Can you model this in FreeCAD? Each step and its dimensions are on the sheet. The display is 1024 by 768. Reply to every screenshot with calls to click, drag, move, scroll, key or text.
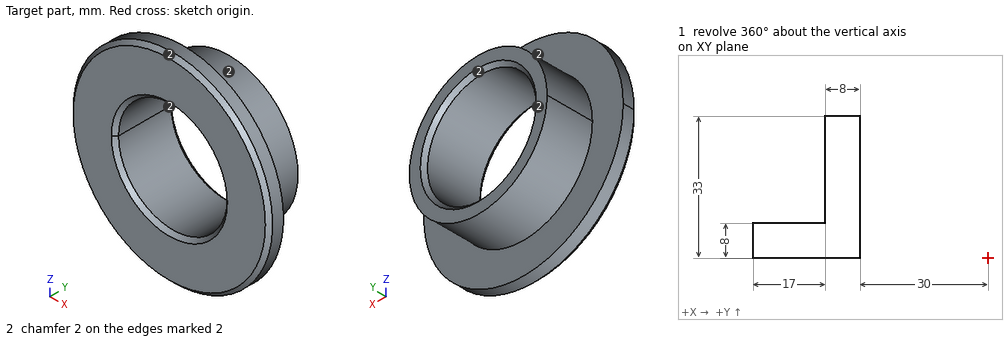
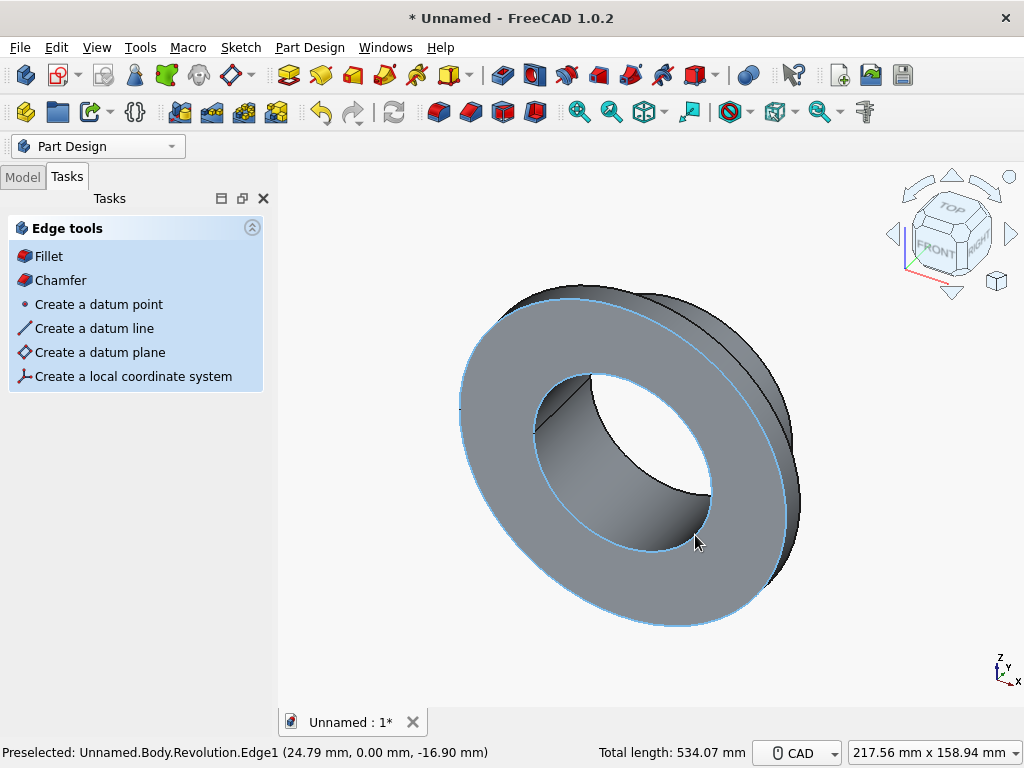
key(0)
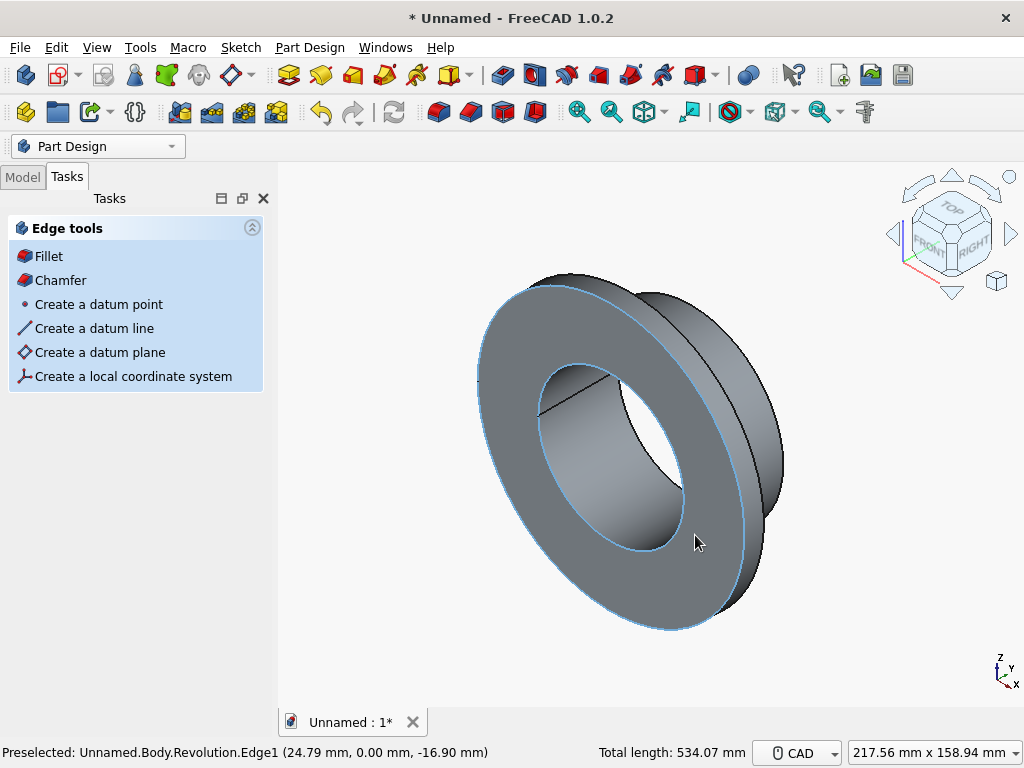
key(2)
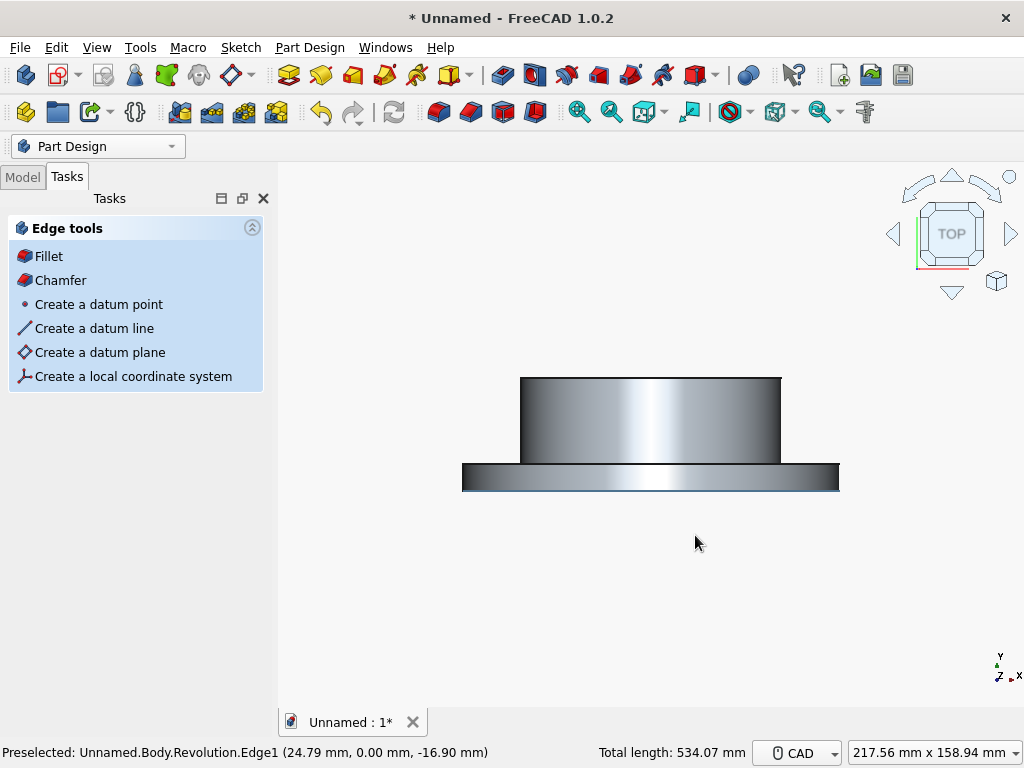
key(1)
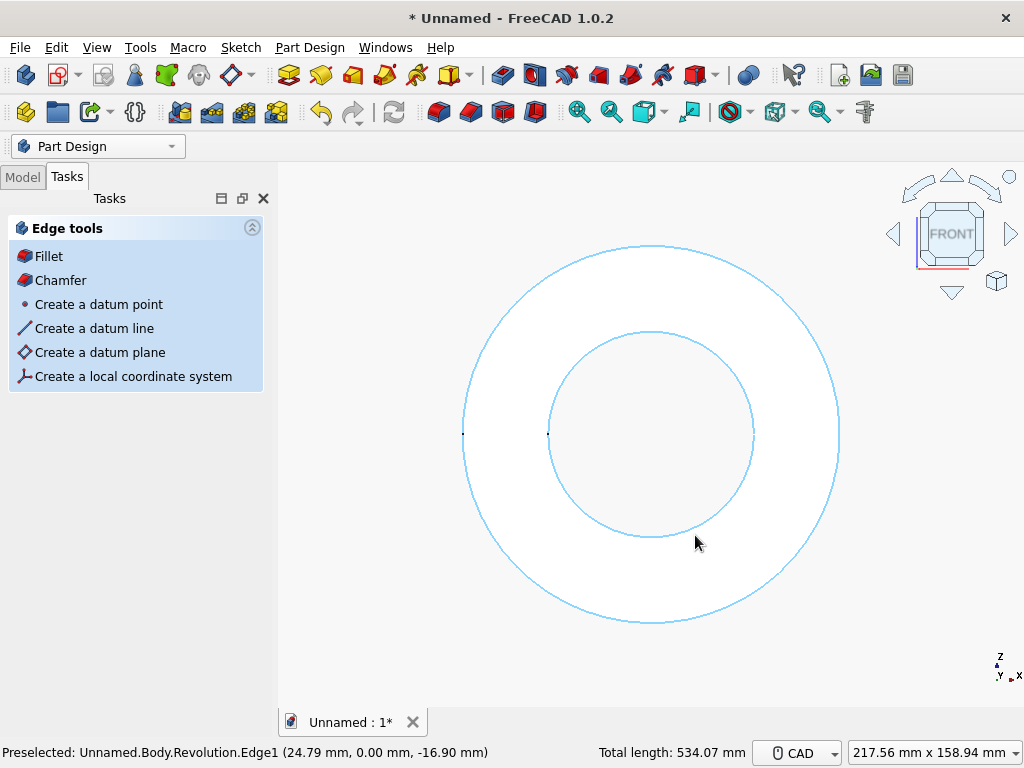
key(3)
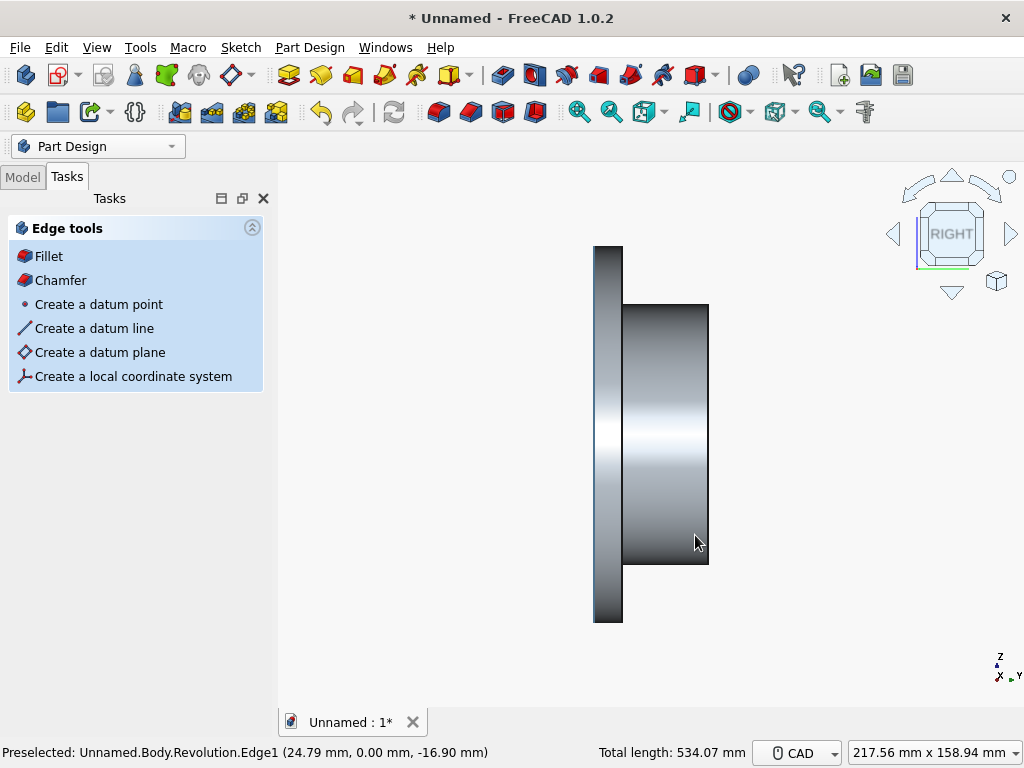
key(5)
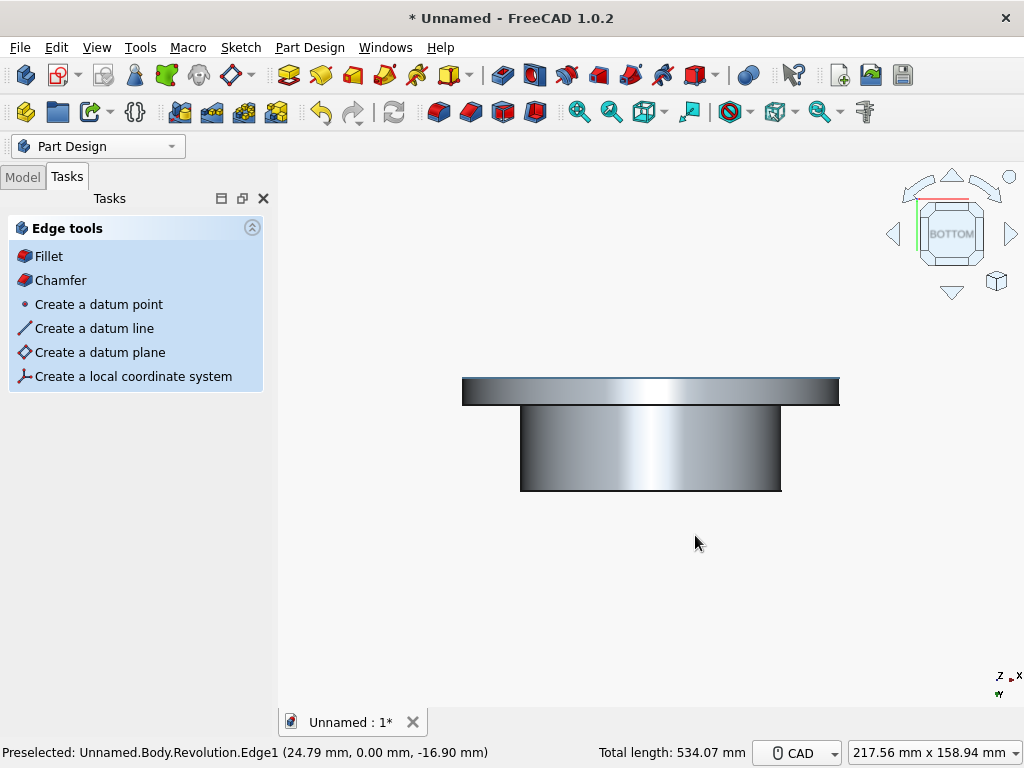
key(4)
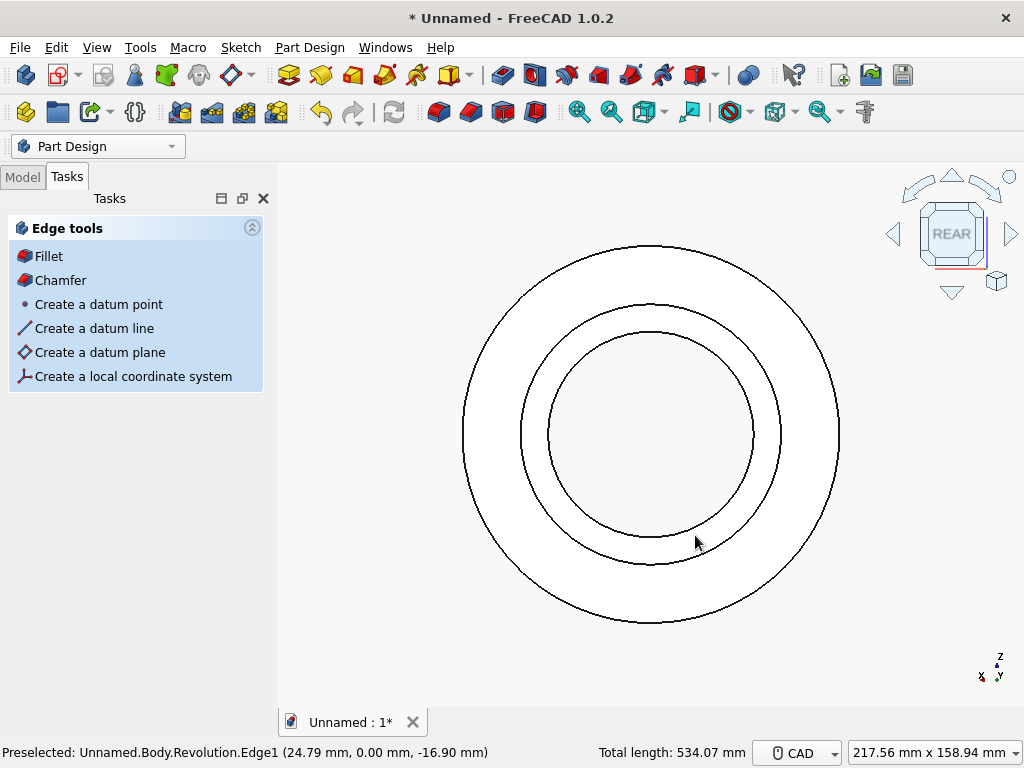
click(548, 433, ctrl)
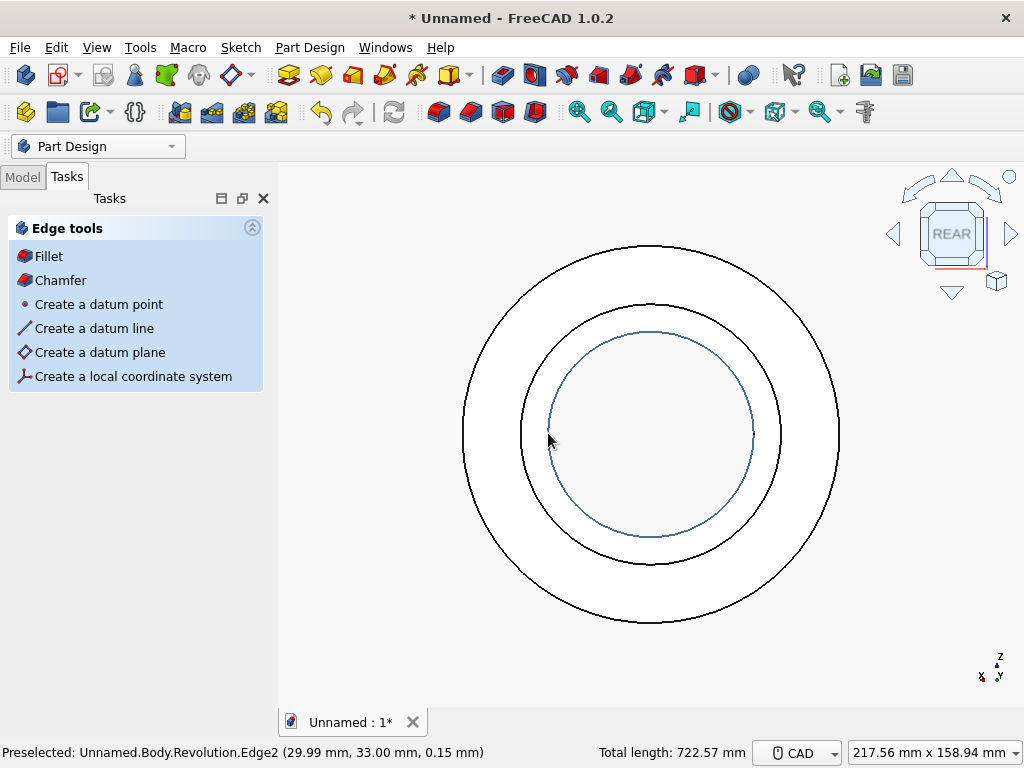
click(472, 112)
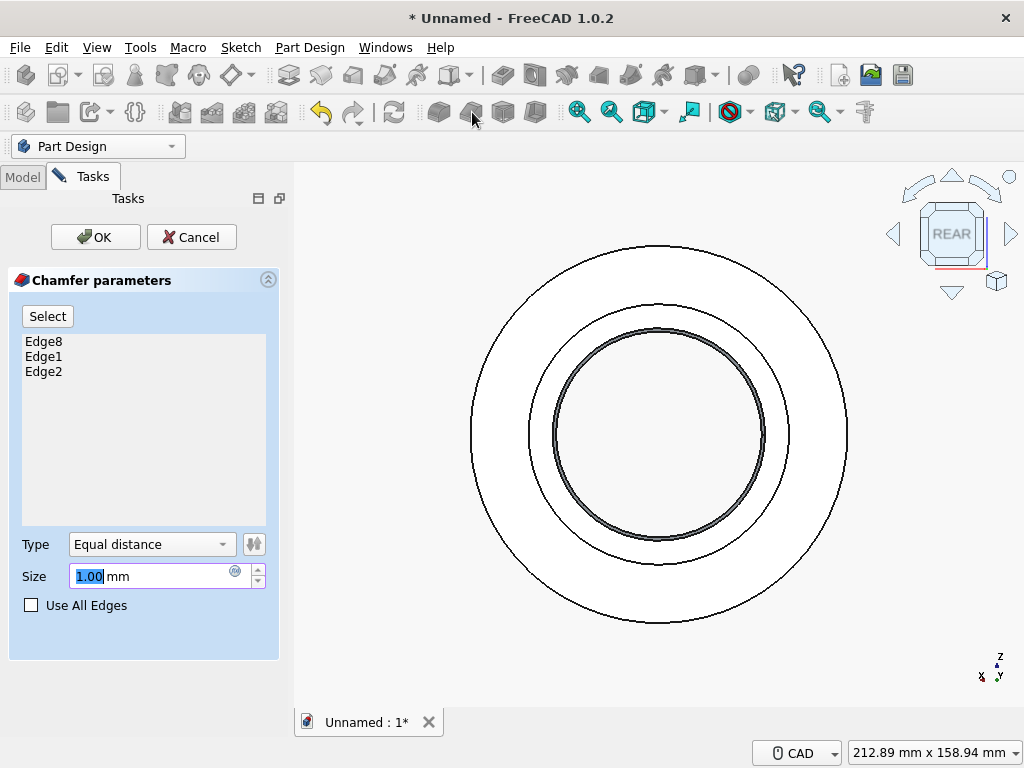
text(2)
key(Tab)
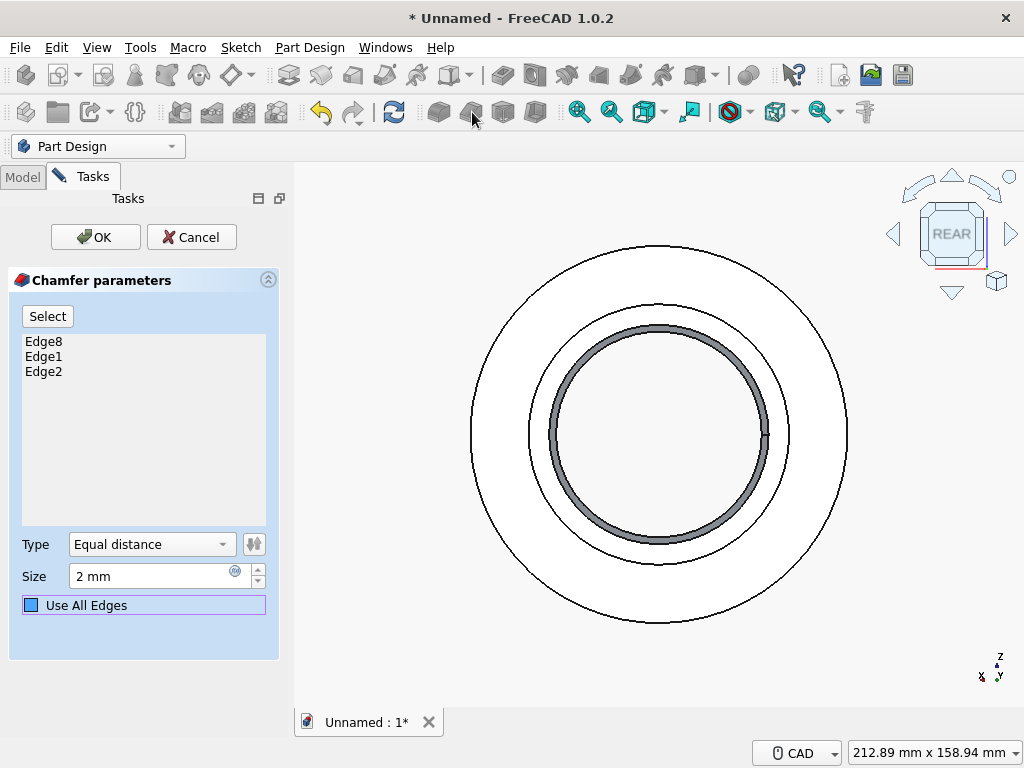
click(96, 237)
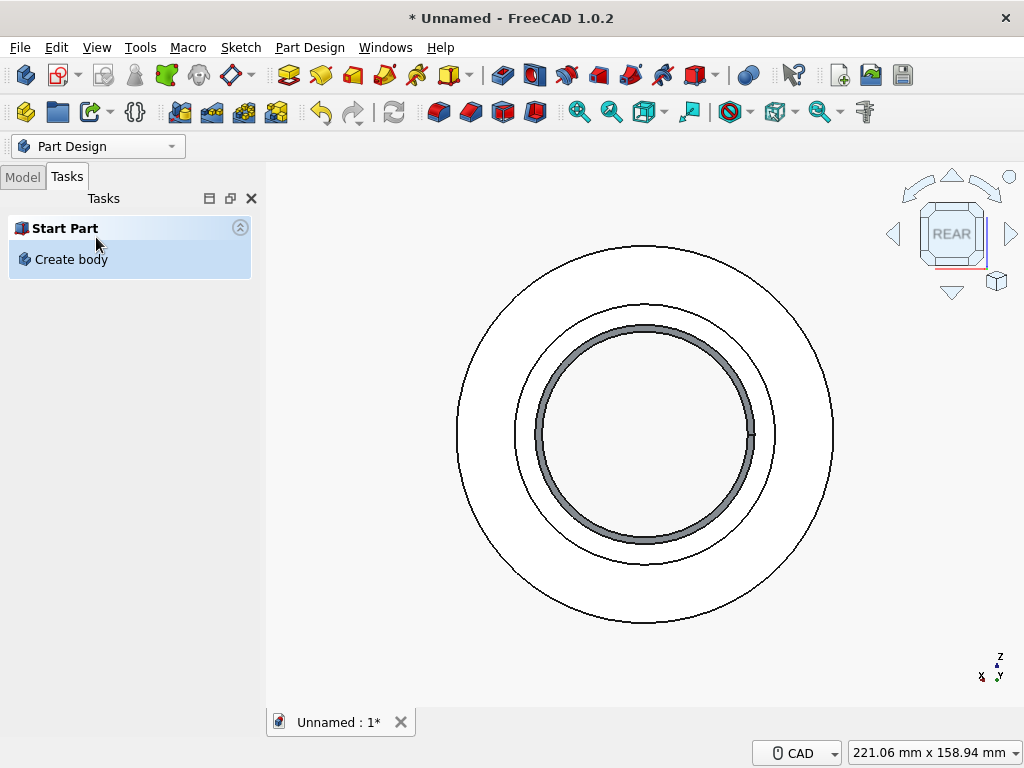
key(0)